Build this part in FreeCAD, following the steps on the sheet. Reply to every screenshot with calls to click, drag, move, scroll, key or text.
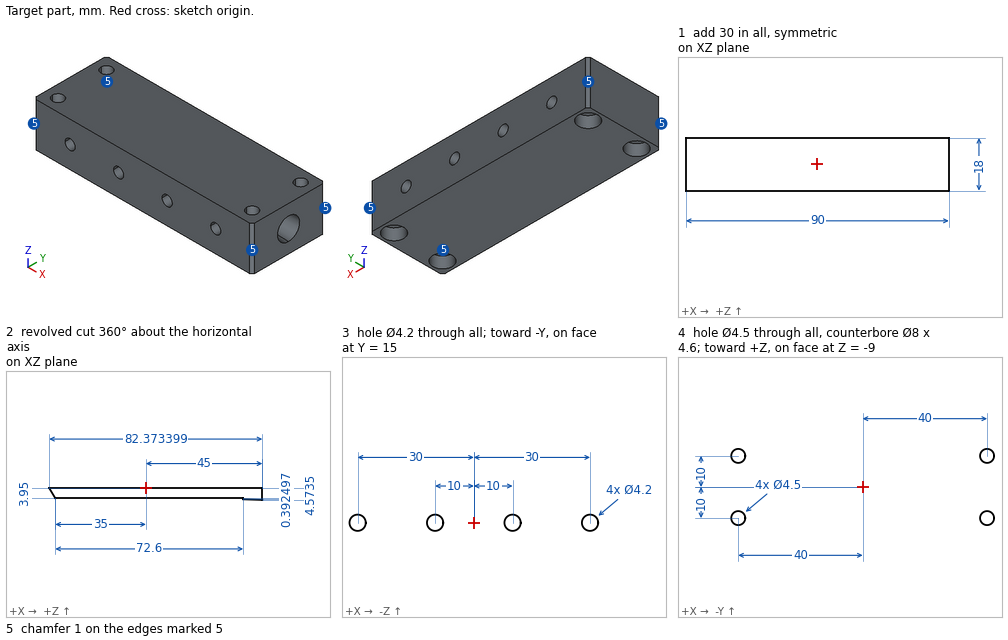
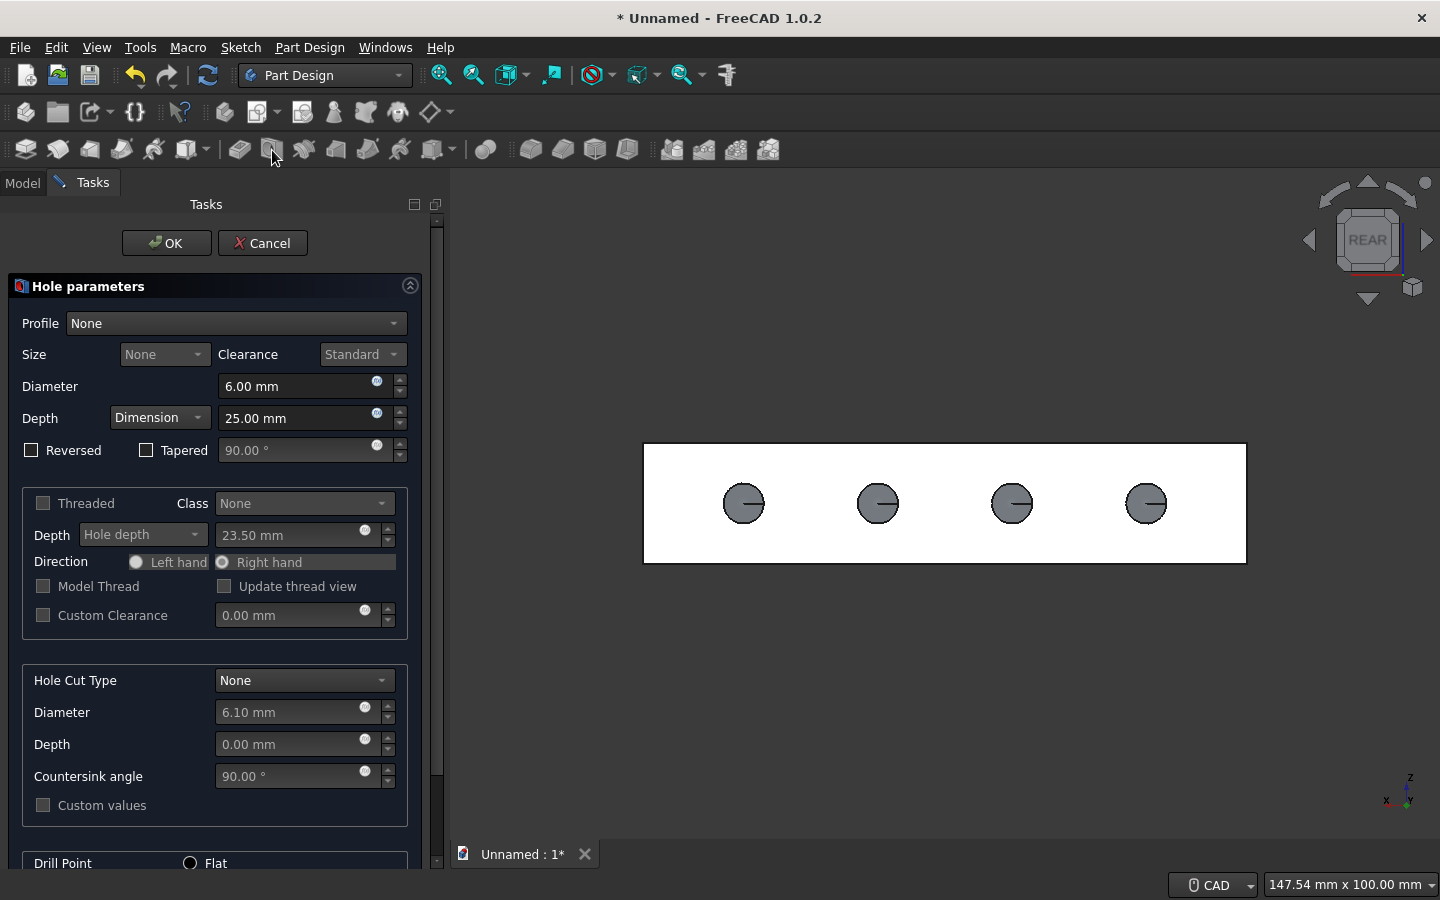
triple_click(305, 386)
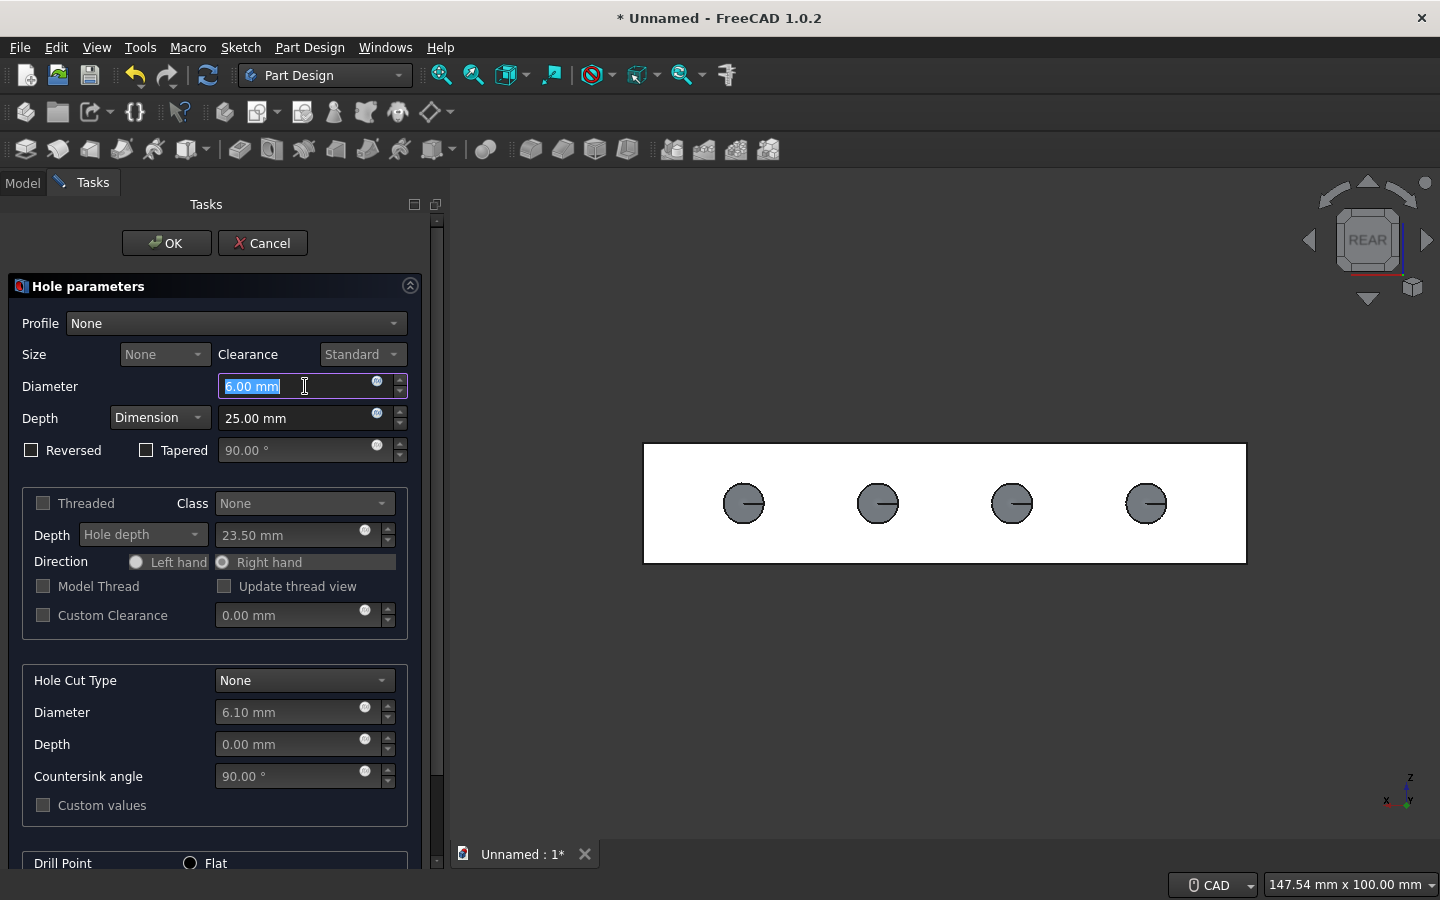
text(4.2)
key(Tab)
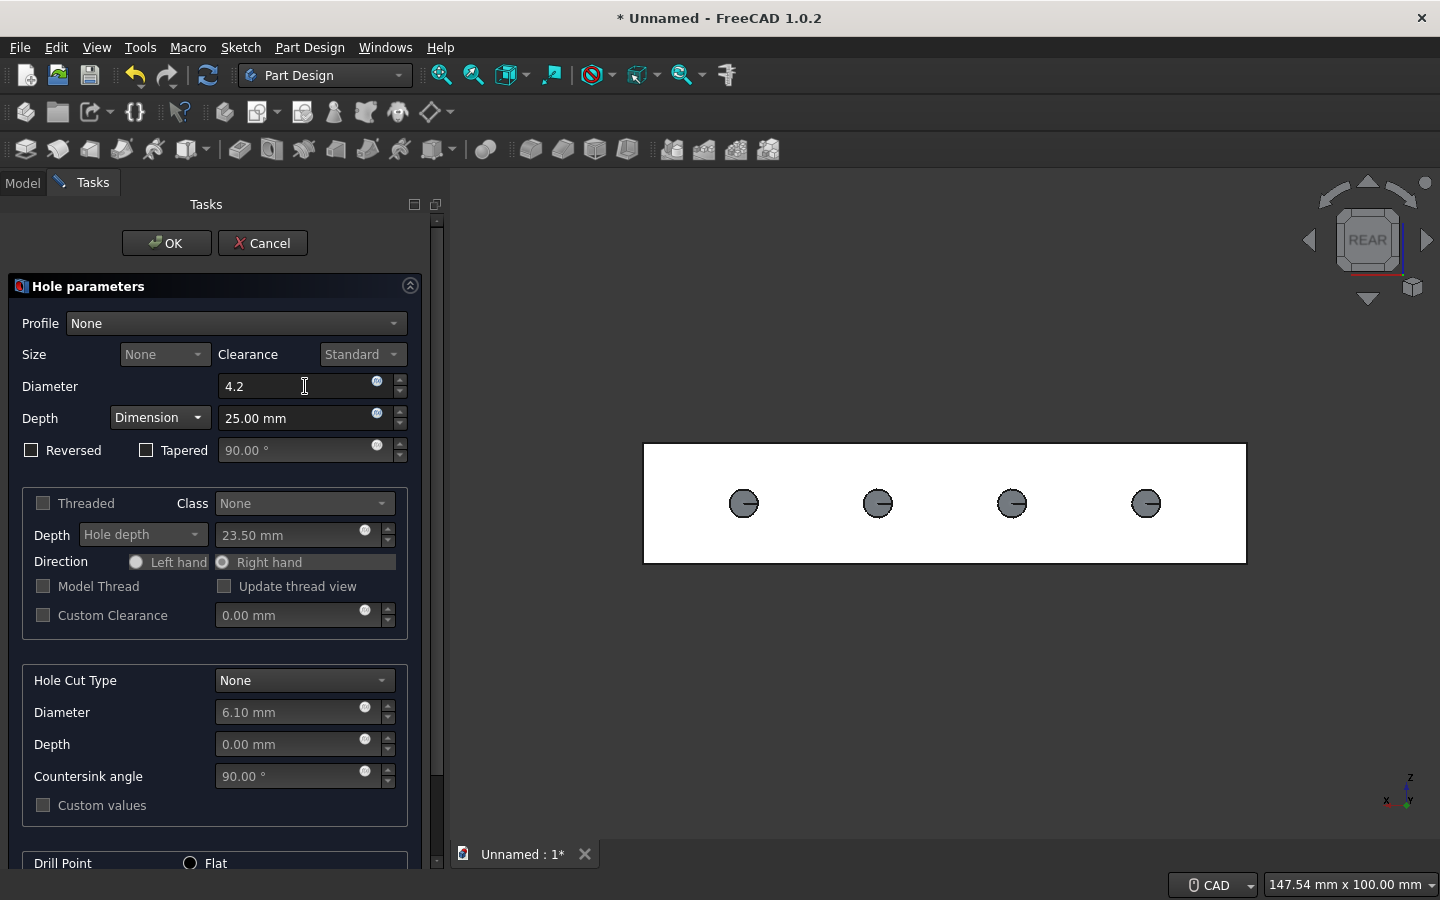
click(161, 418)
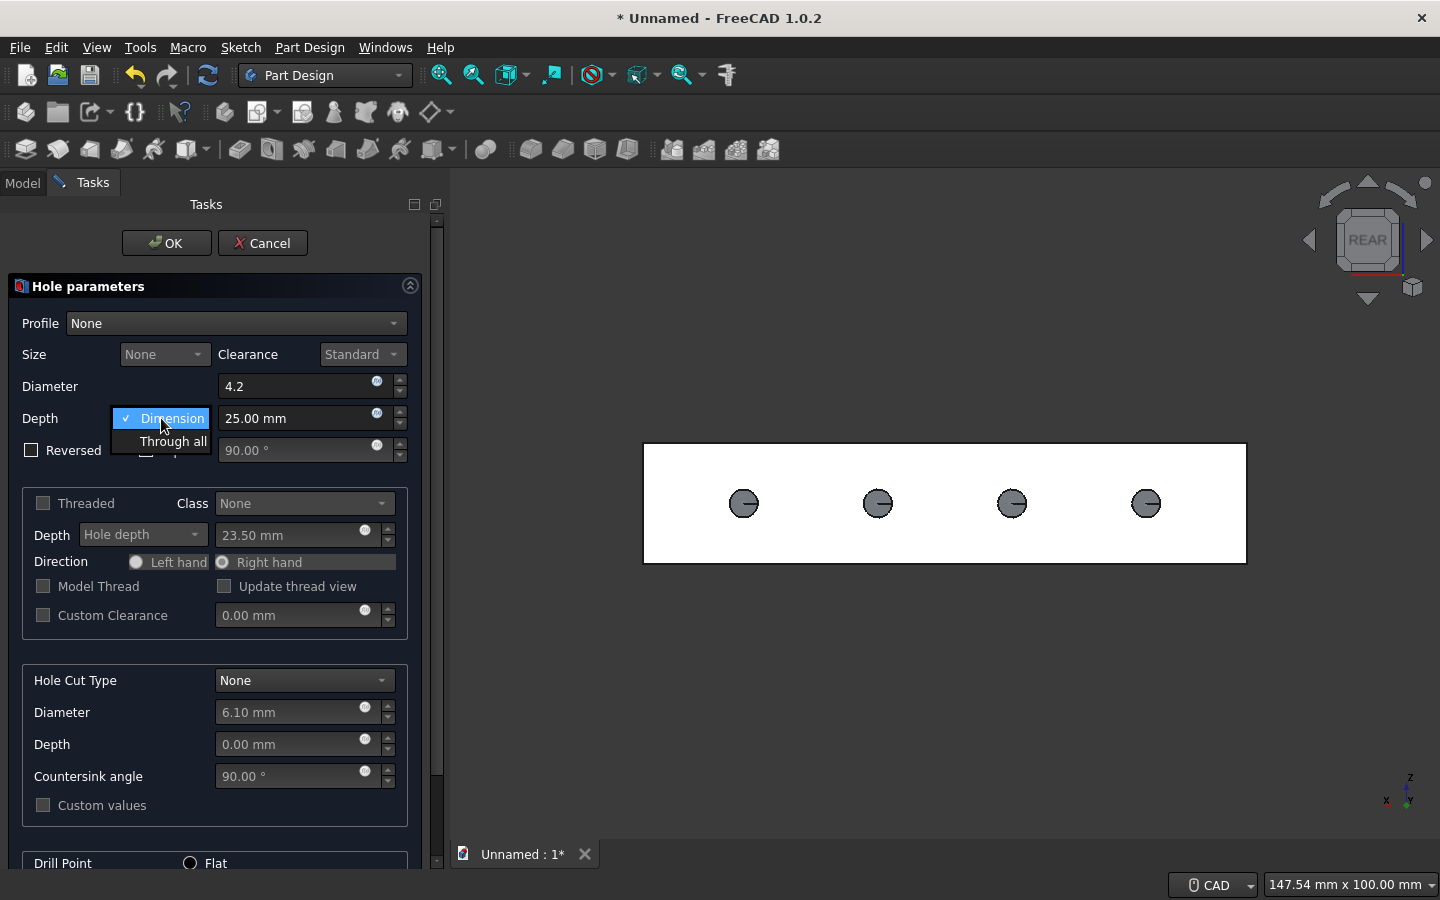
click(160, 442)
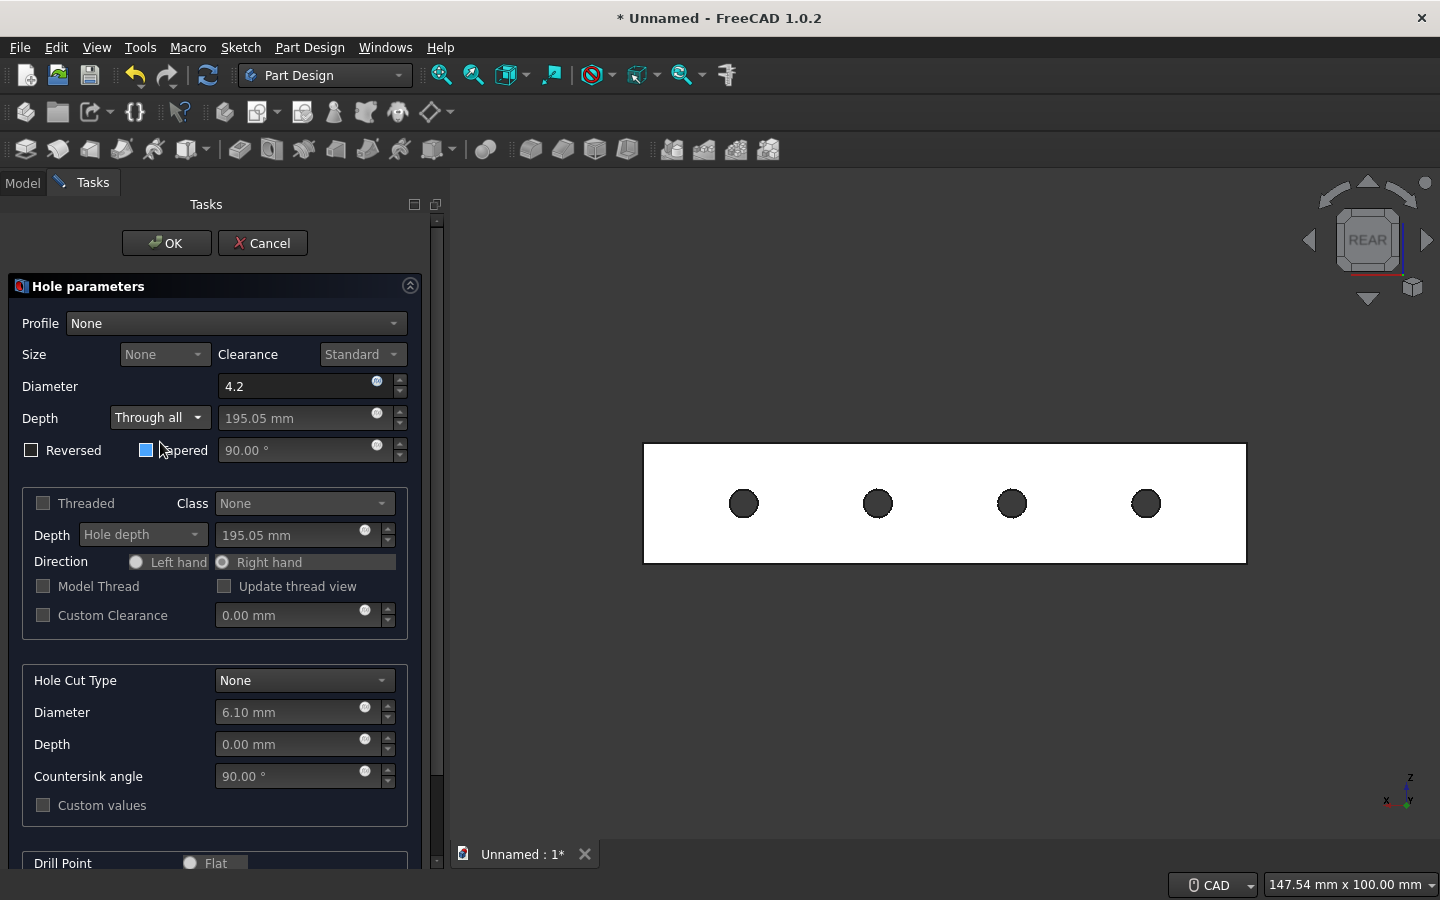
click(167, 243)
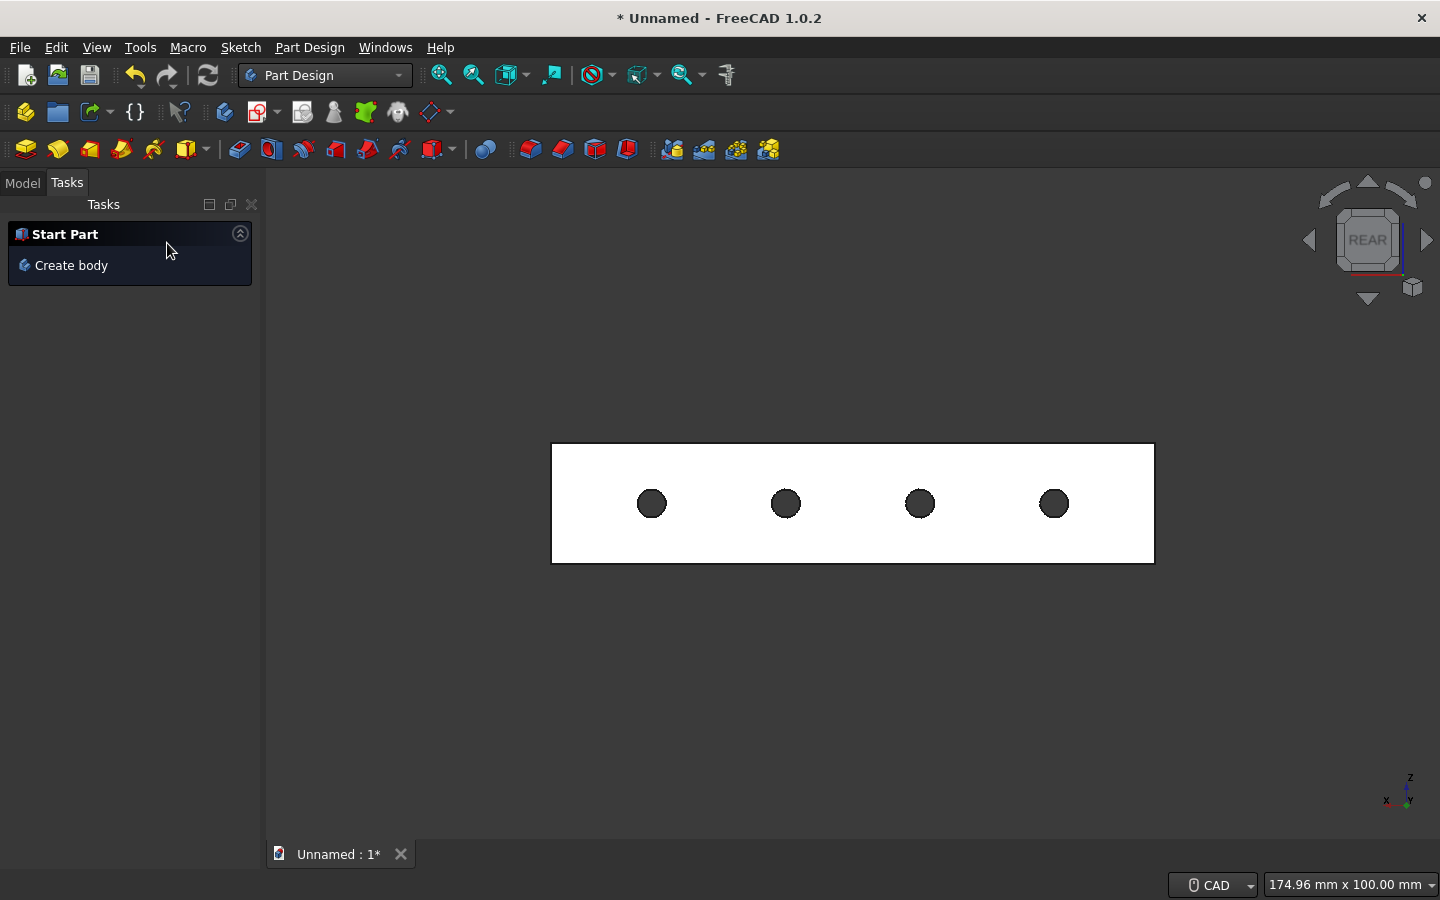
key(5)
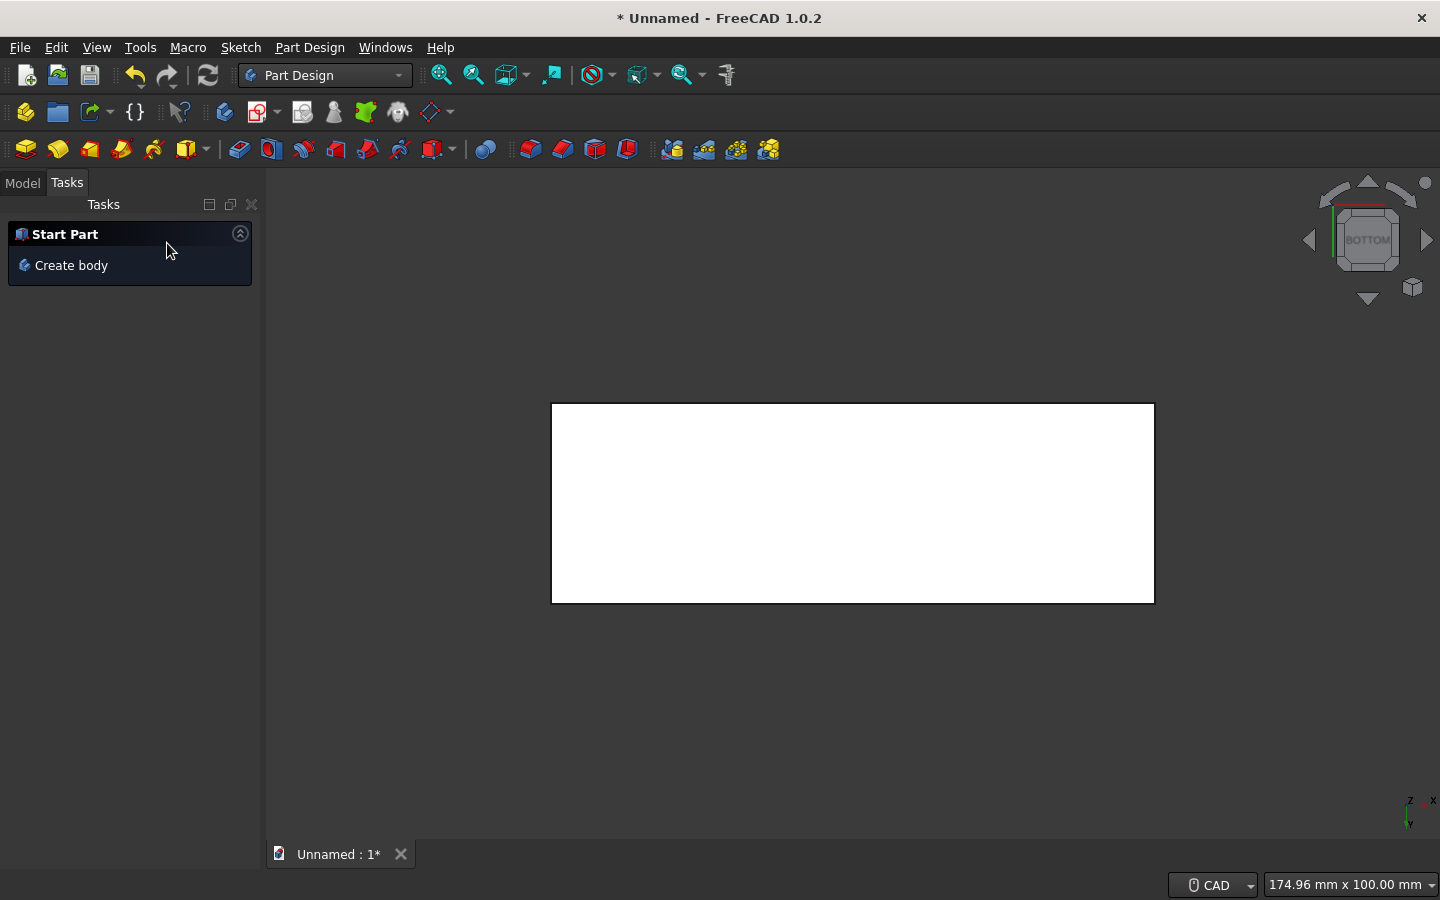
click(1026, 503)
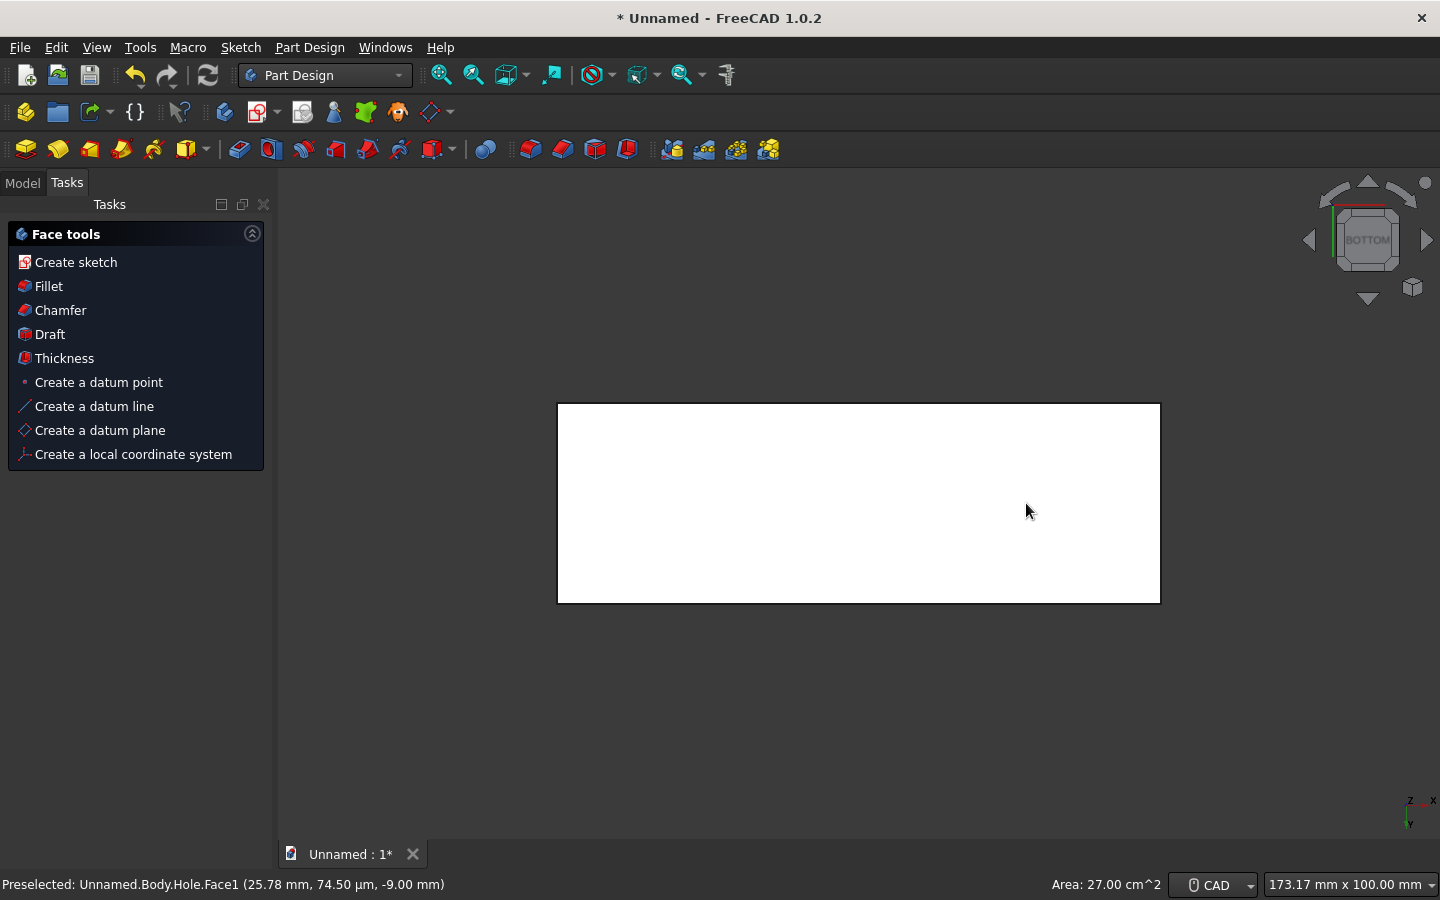
click(258, 112)